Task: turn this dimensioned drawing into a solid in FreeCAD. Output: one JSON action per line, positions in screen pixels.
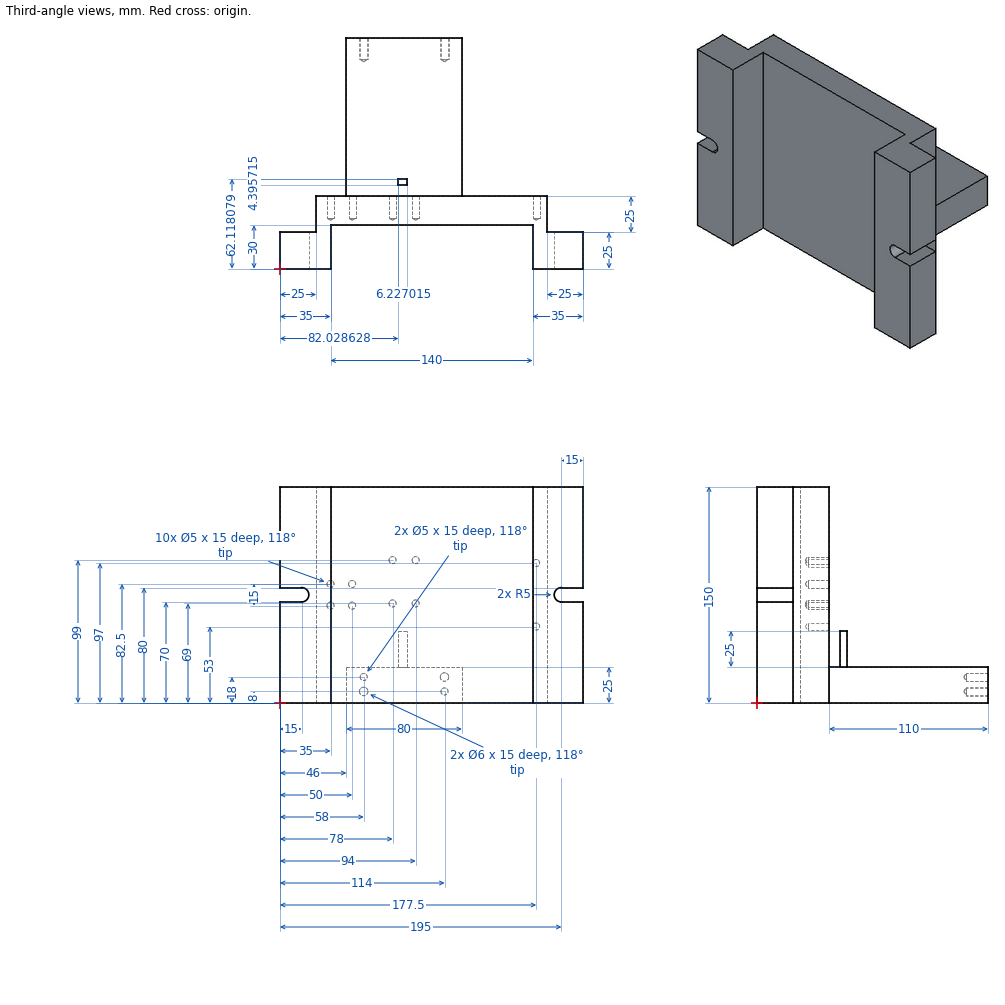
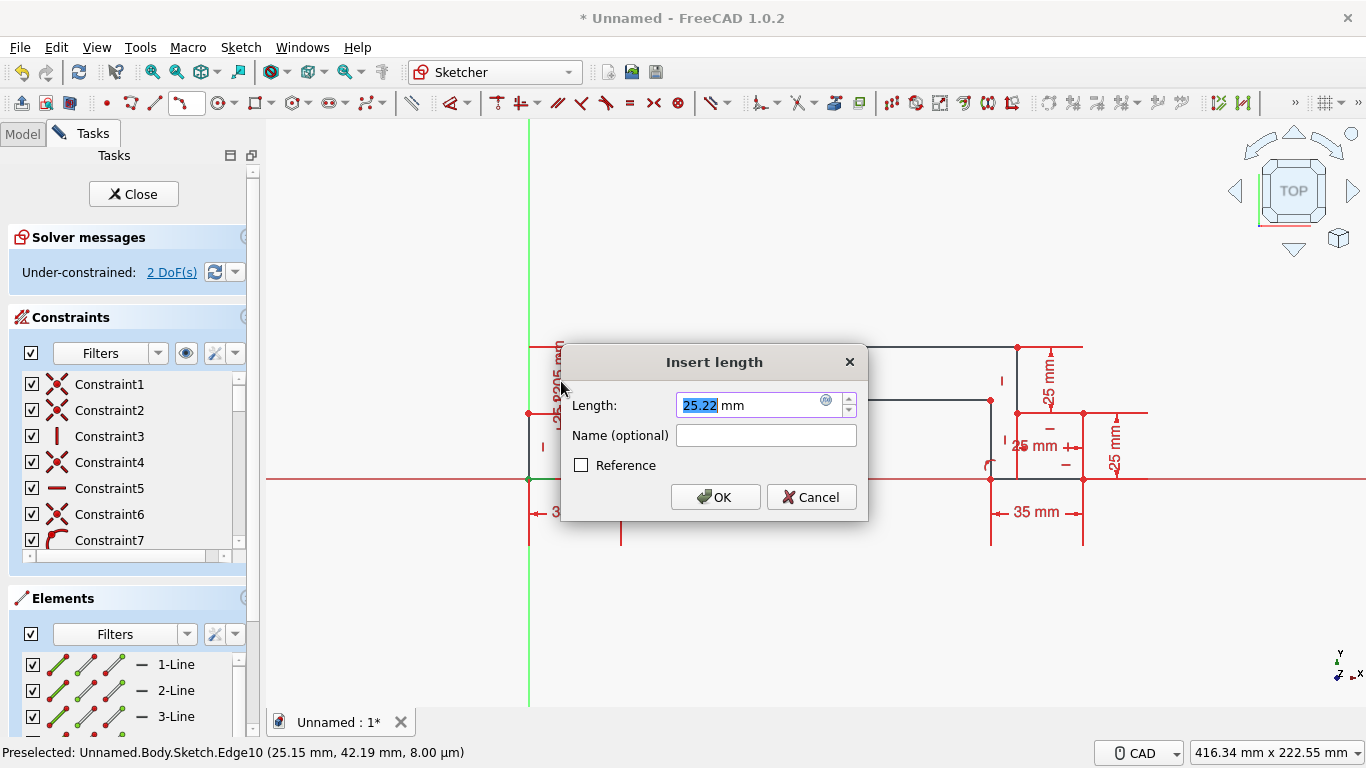
{"action": "type", "text": "25"}
{"action": "key", "text": "Return"}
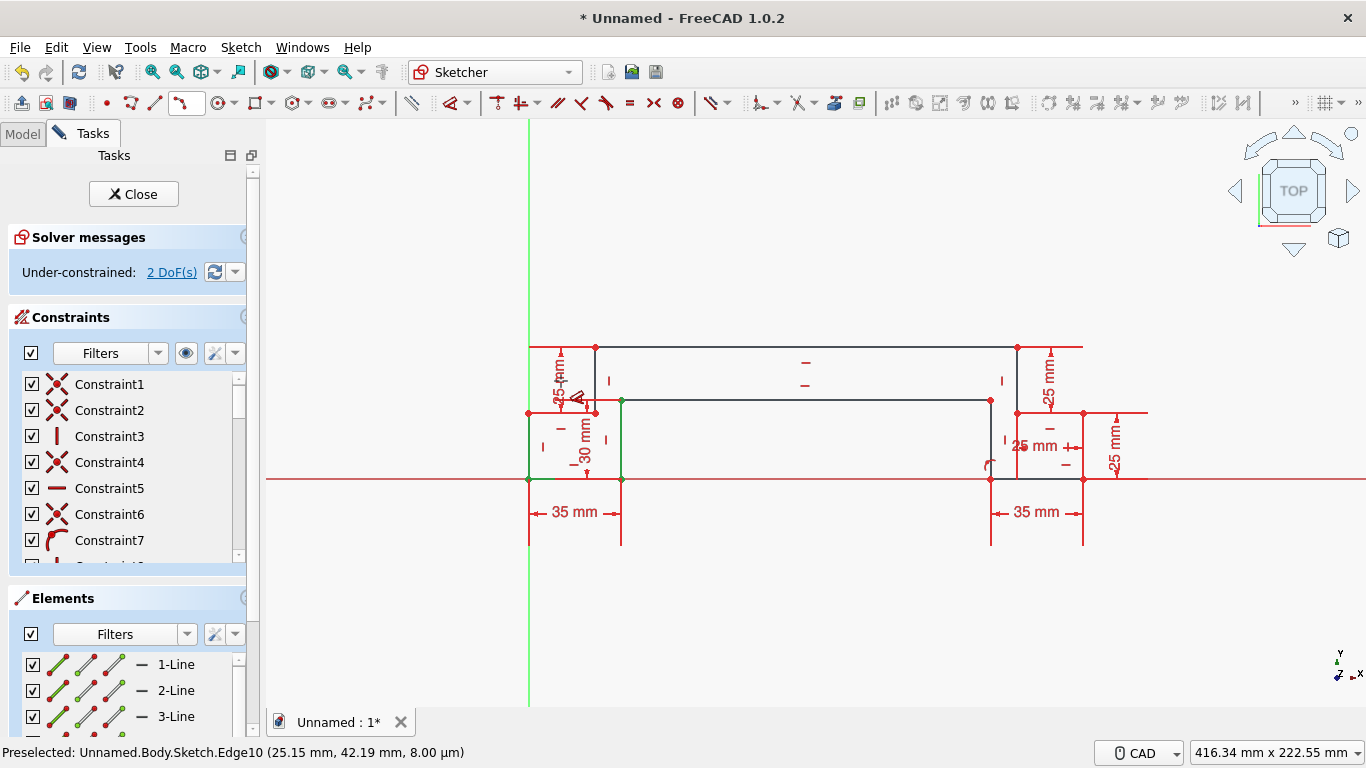
{"action": "left_click", "coordinate": [575, 413]}
{"action": "left_click", "coordinate": [562, 355]}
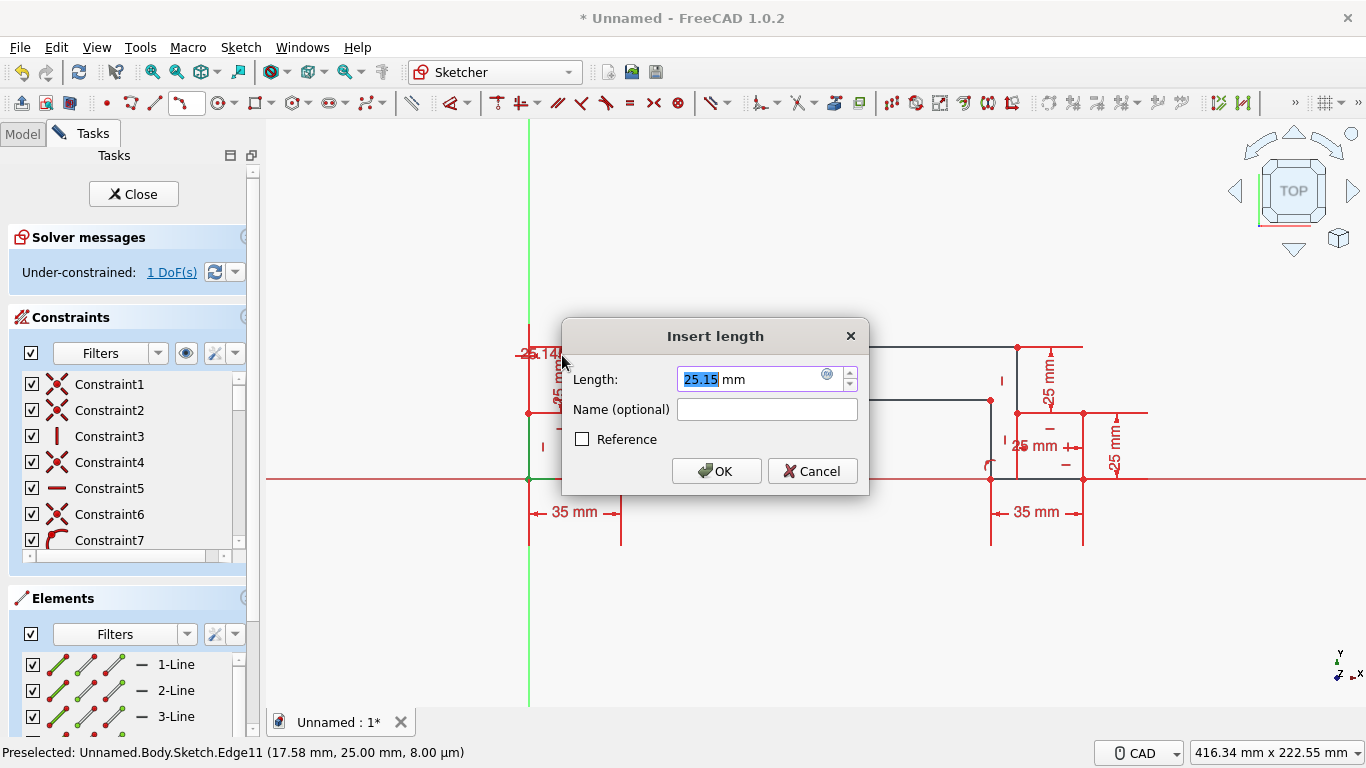
{"action": "type", "text": "25"}
{"action": "key", "text": "Return"}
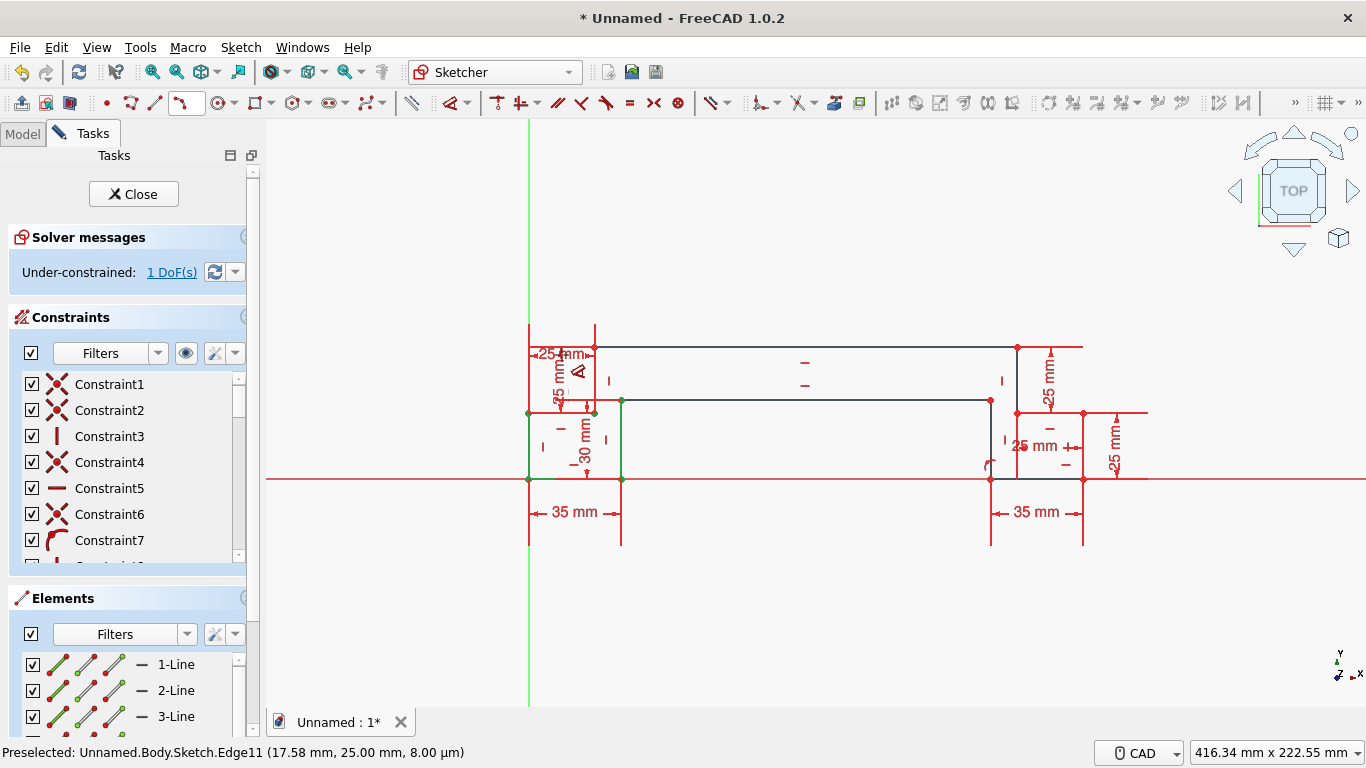
{"action": "left_click", "coordinate": [732, 400]}
{"action": "left_click", "coordinate": [806, 366]}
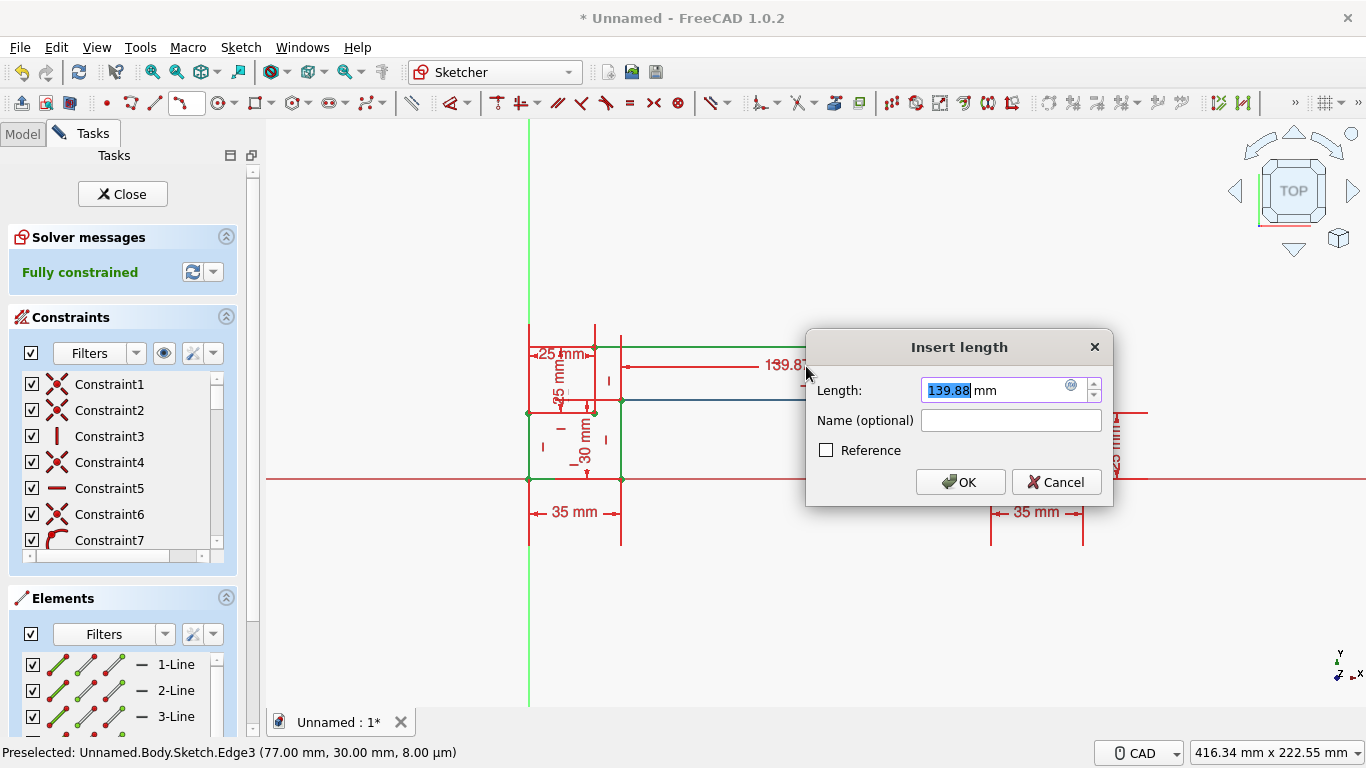
{"action": "type", "text": "140"}
{"action": "key", "text": "Return"}
{"action": "key", "text": "Escape"}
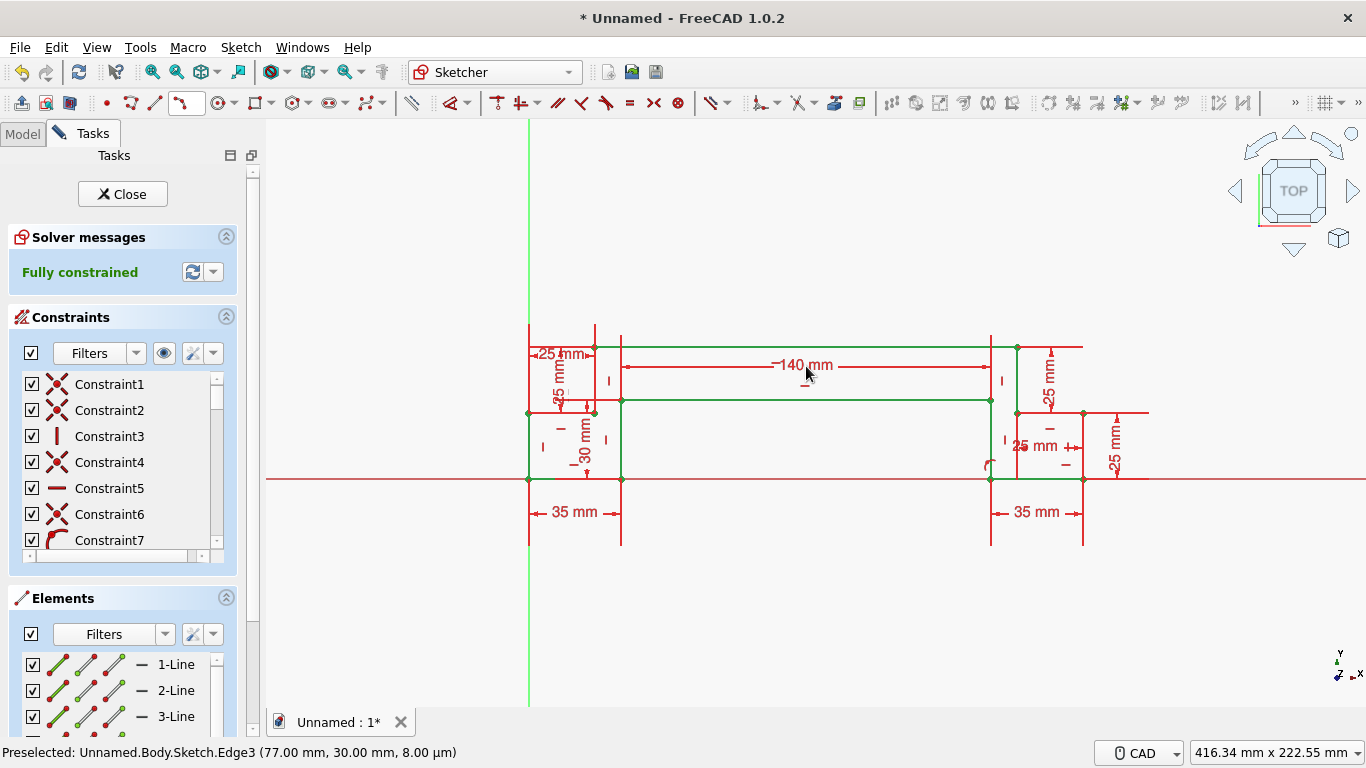
{"action": "left_click", "coordinate": [123, 194]}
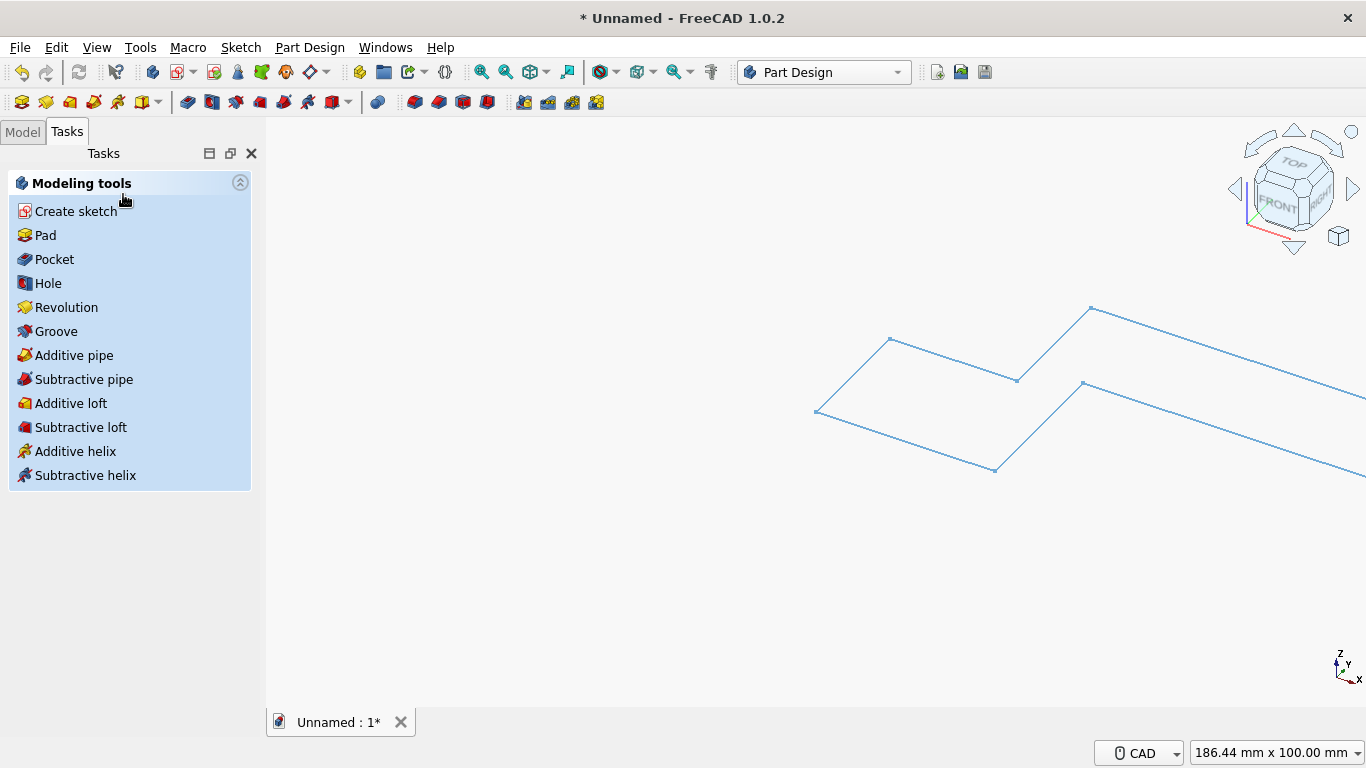
{"action": "left_click", "coordinate": [22, 102]}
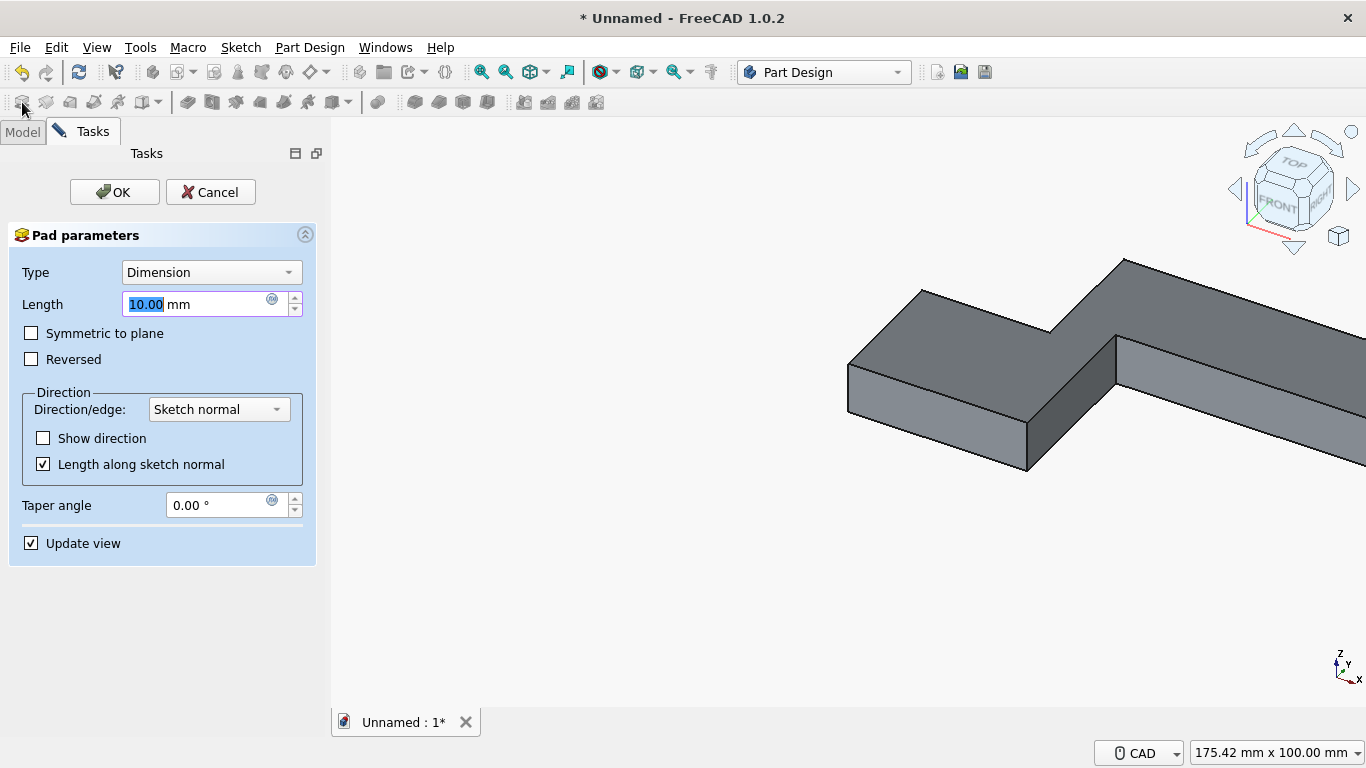
{"action": "type", "text": "150"}
{"action": "key", "text": "Tab"}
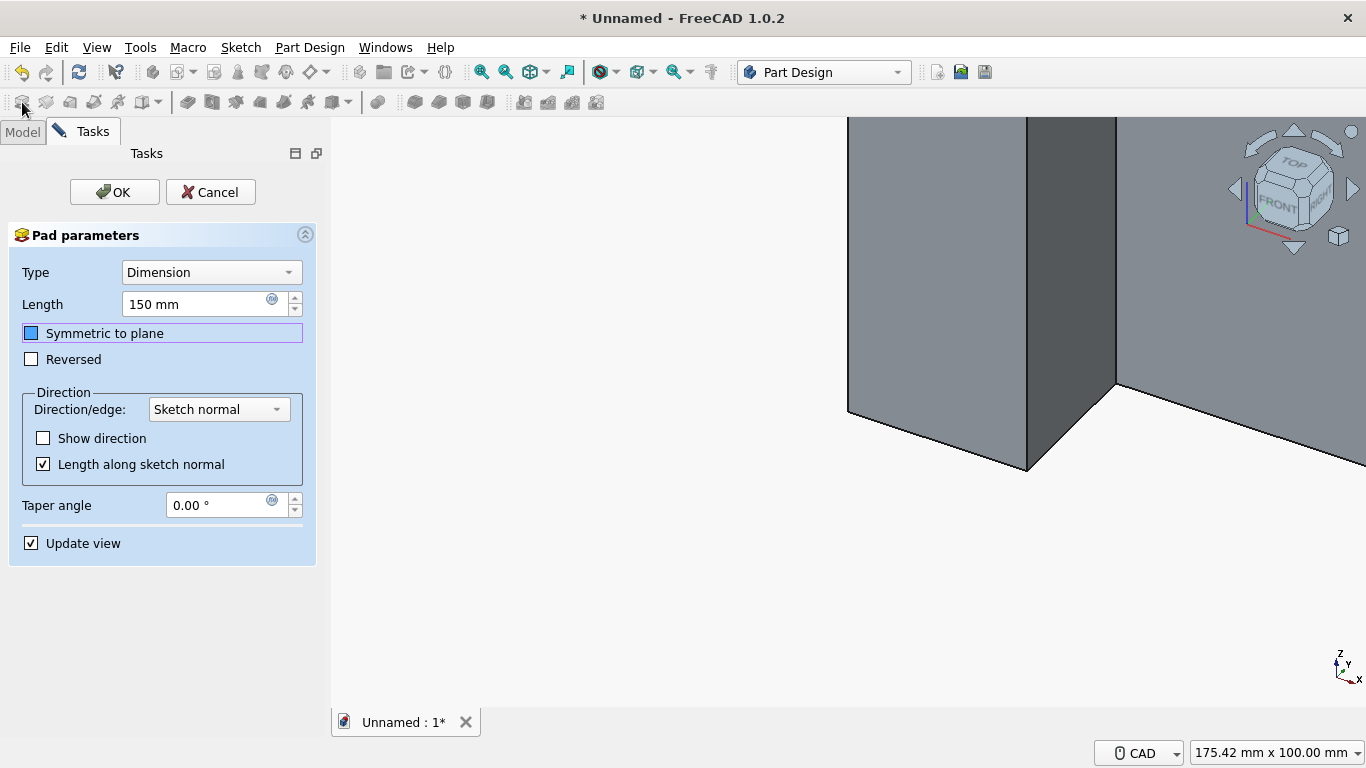
{"action": "left_click", "coordinate": [115, 192]}